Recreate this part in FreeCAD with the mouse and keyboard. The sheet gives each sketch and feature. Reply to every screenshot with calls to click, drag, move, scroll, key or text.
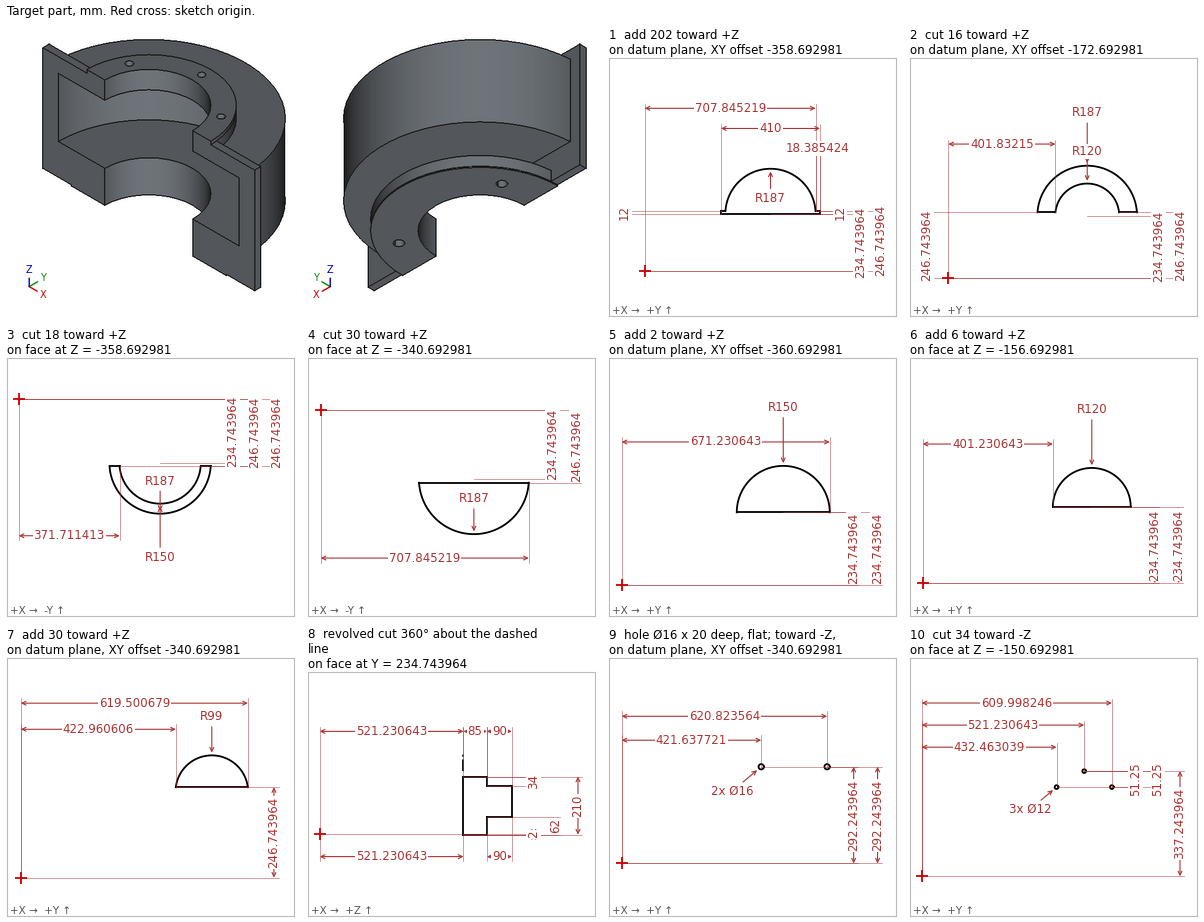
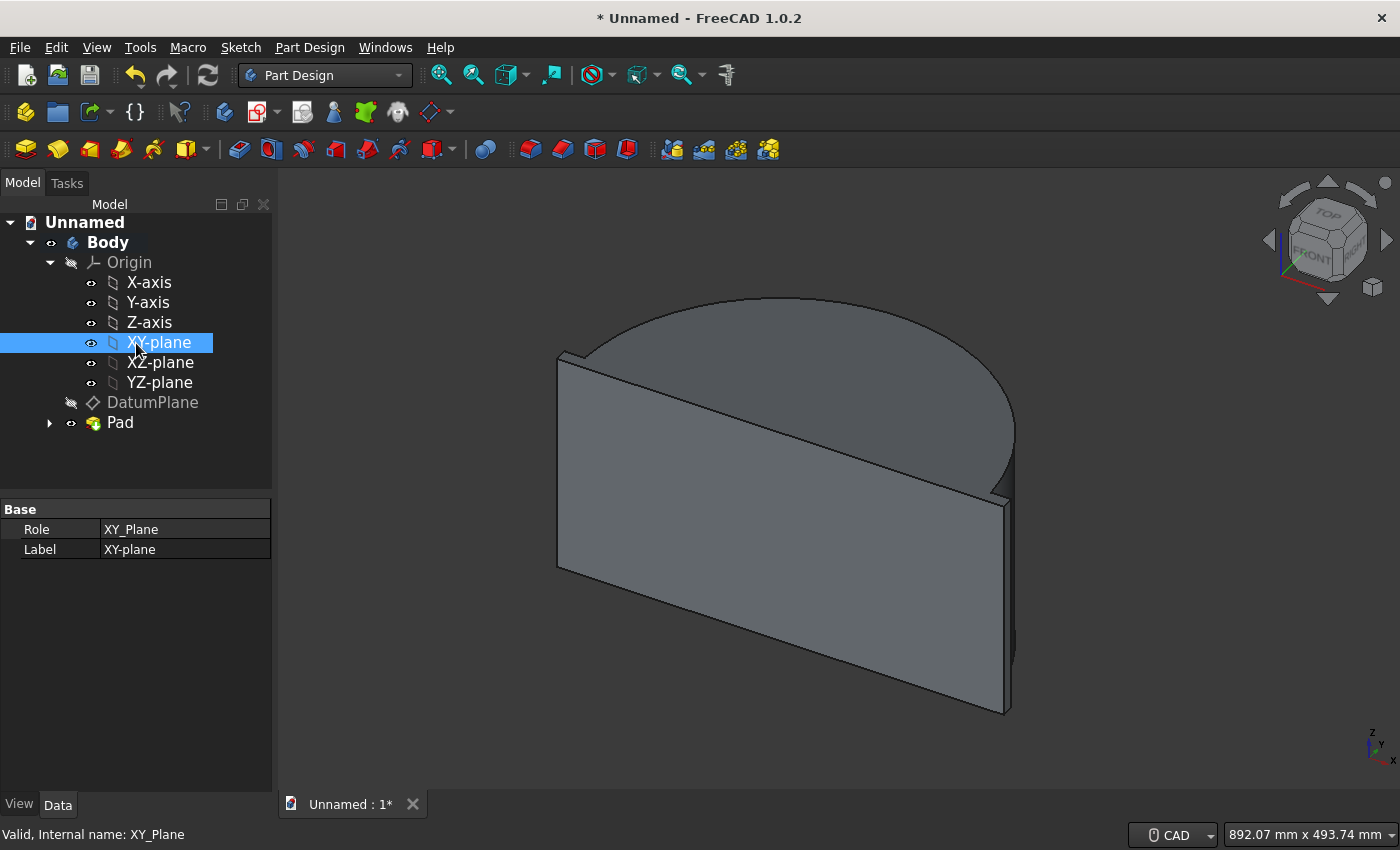
click(430, 112)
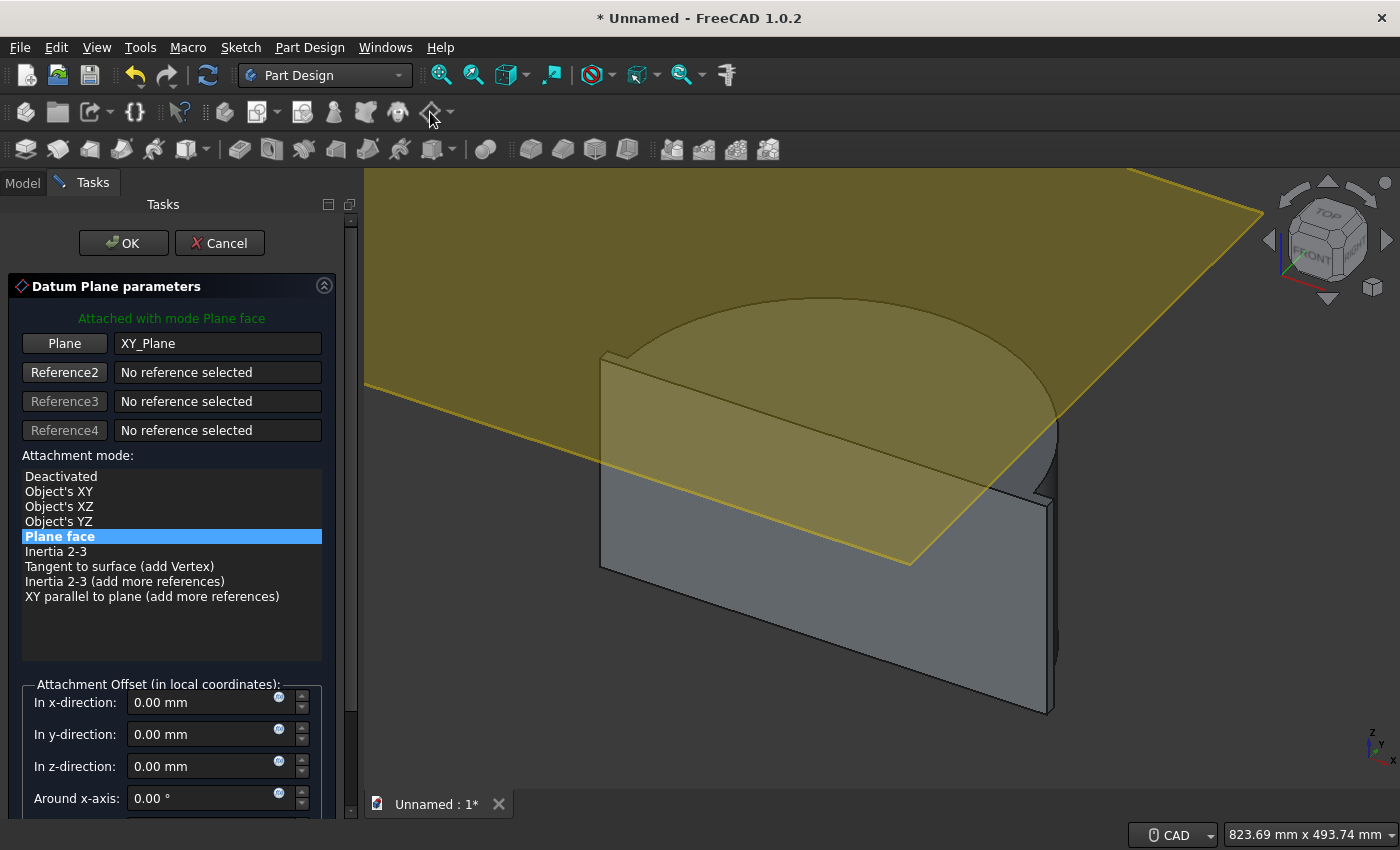
triple_click(210, 766)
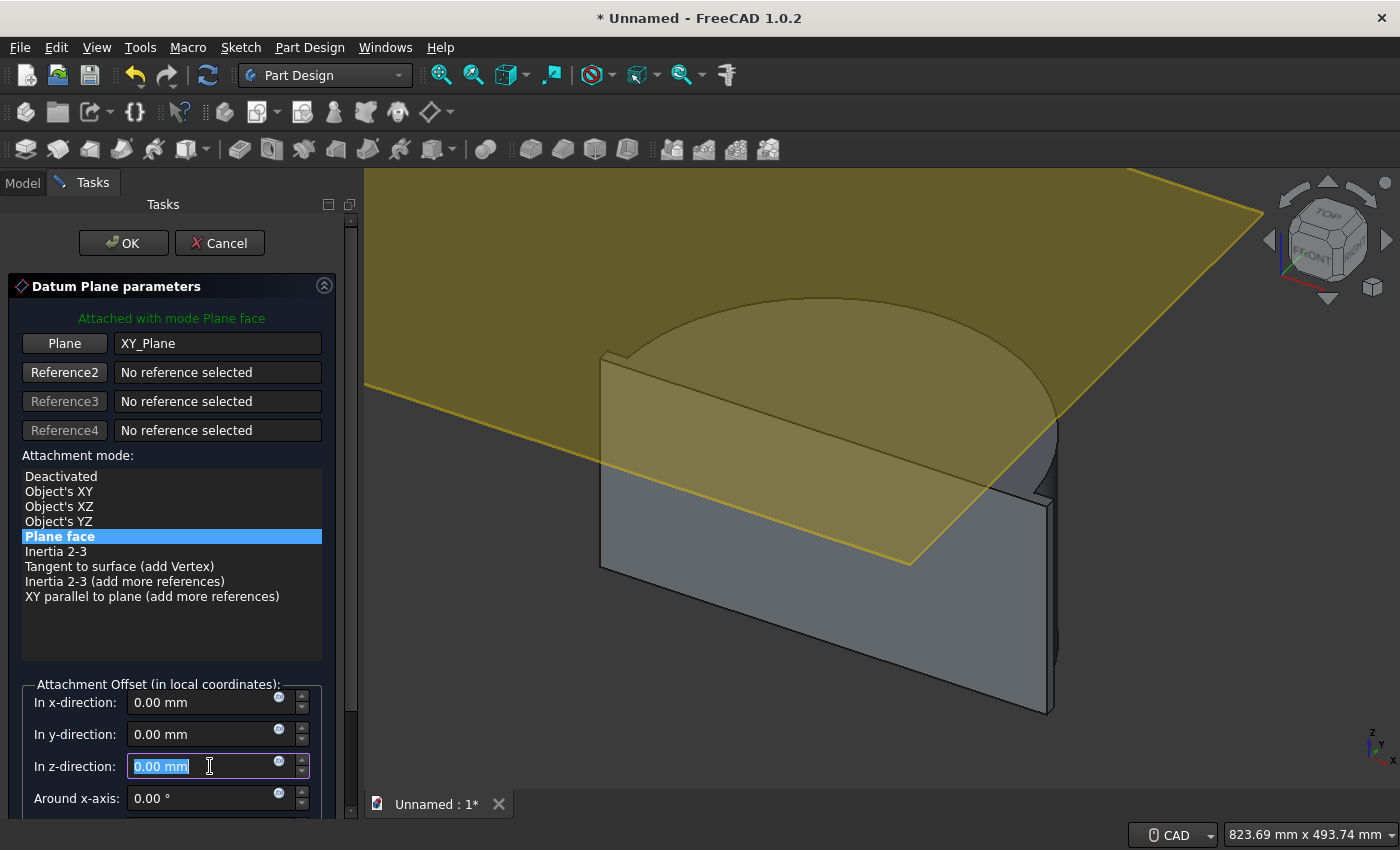
text(-172.692981)
key(Tab)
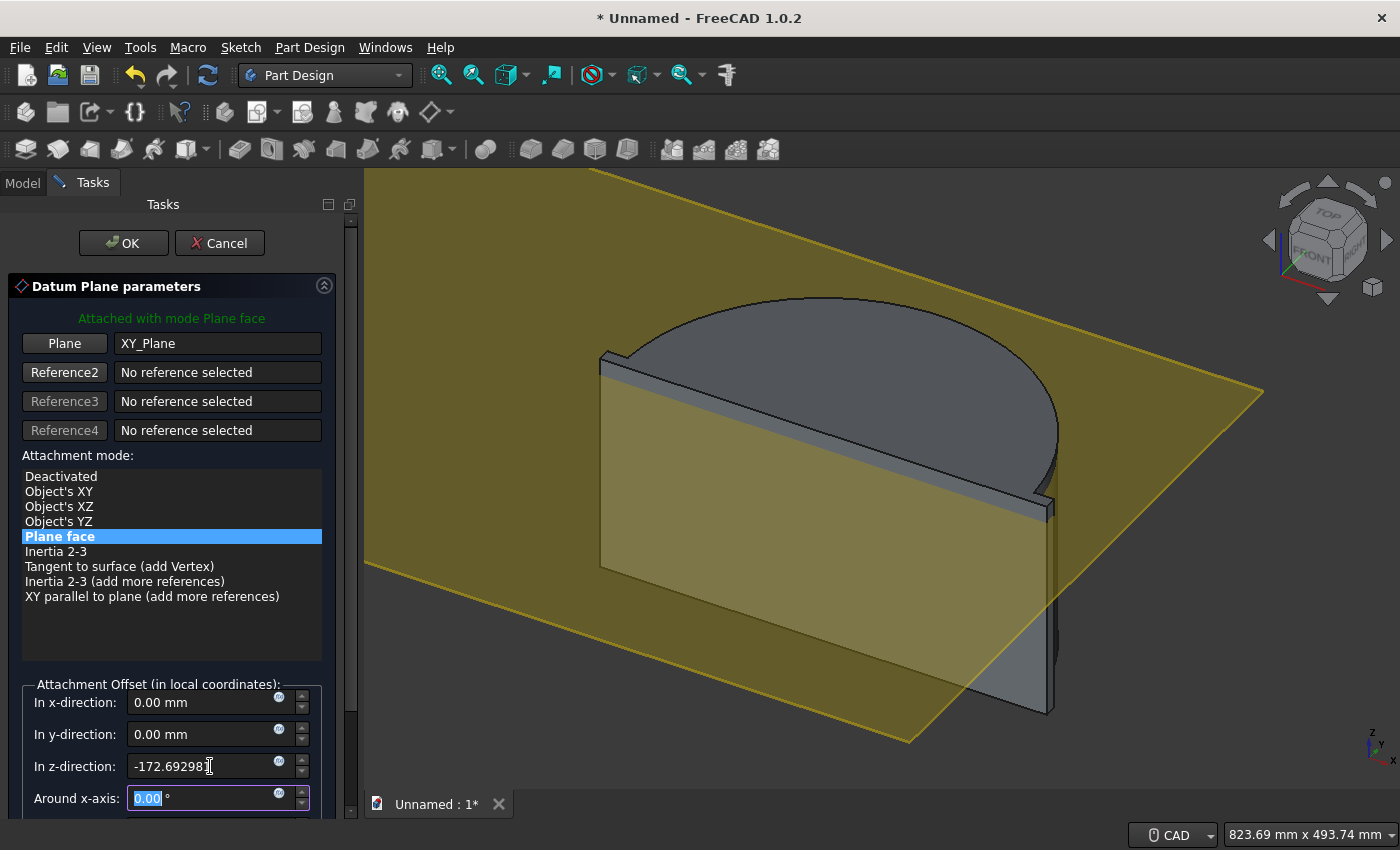
click(124, 243)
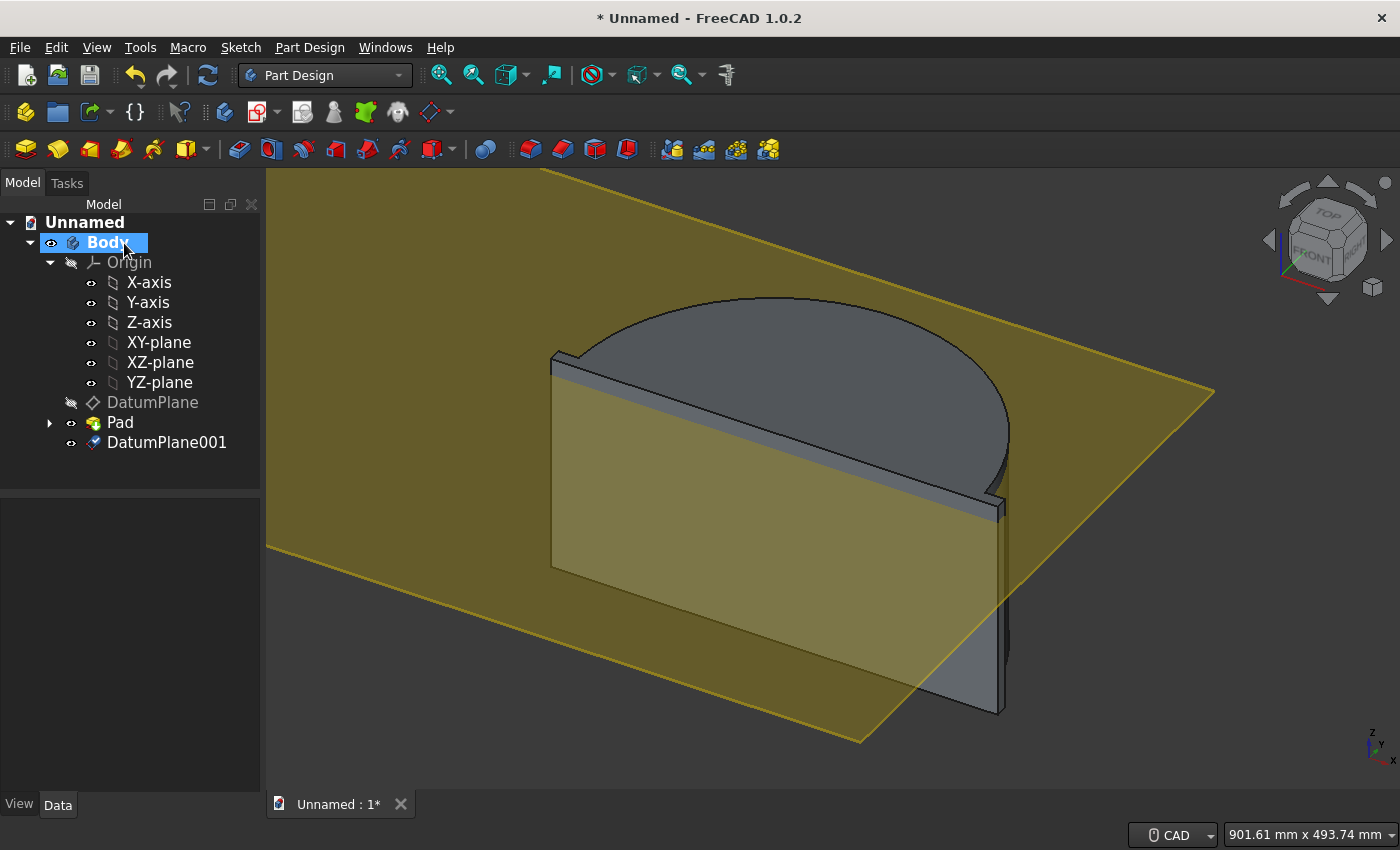
click(116, 443)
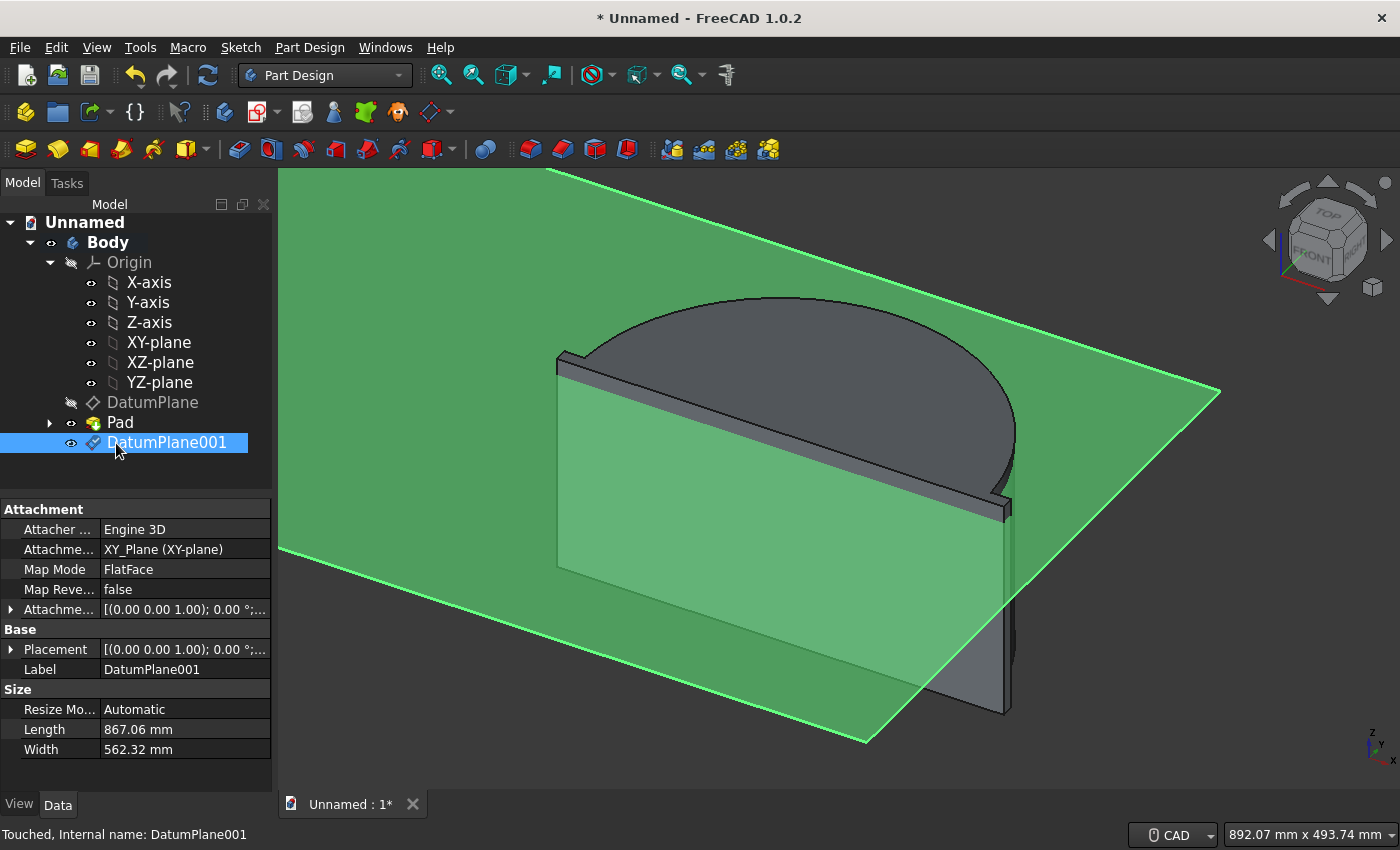
click(258, 112)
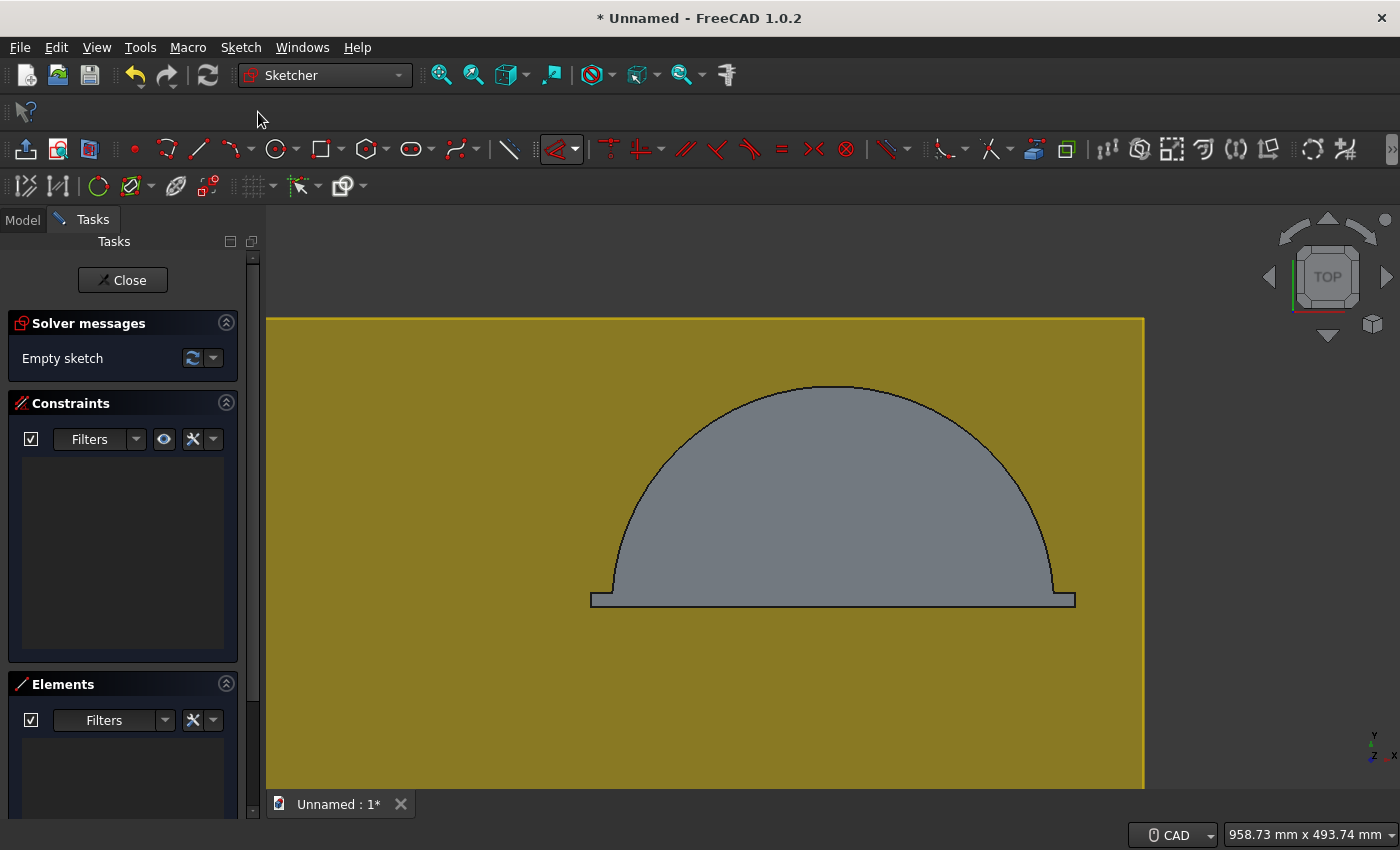
key(q)
key(s)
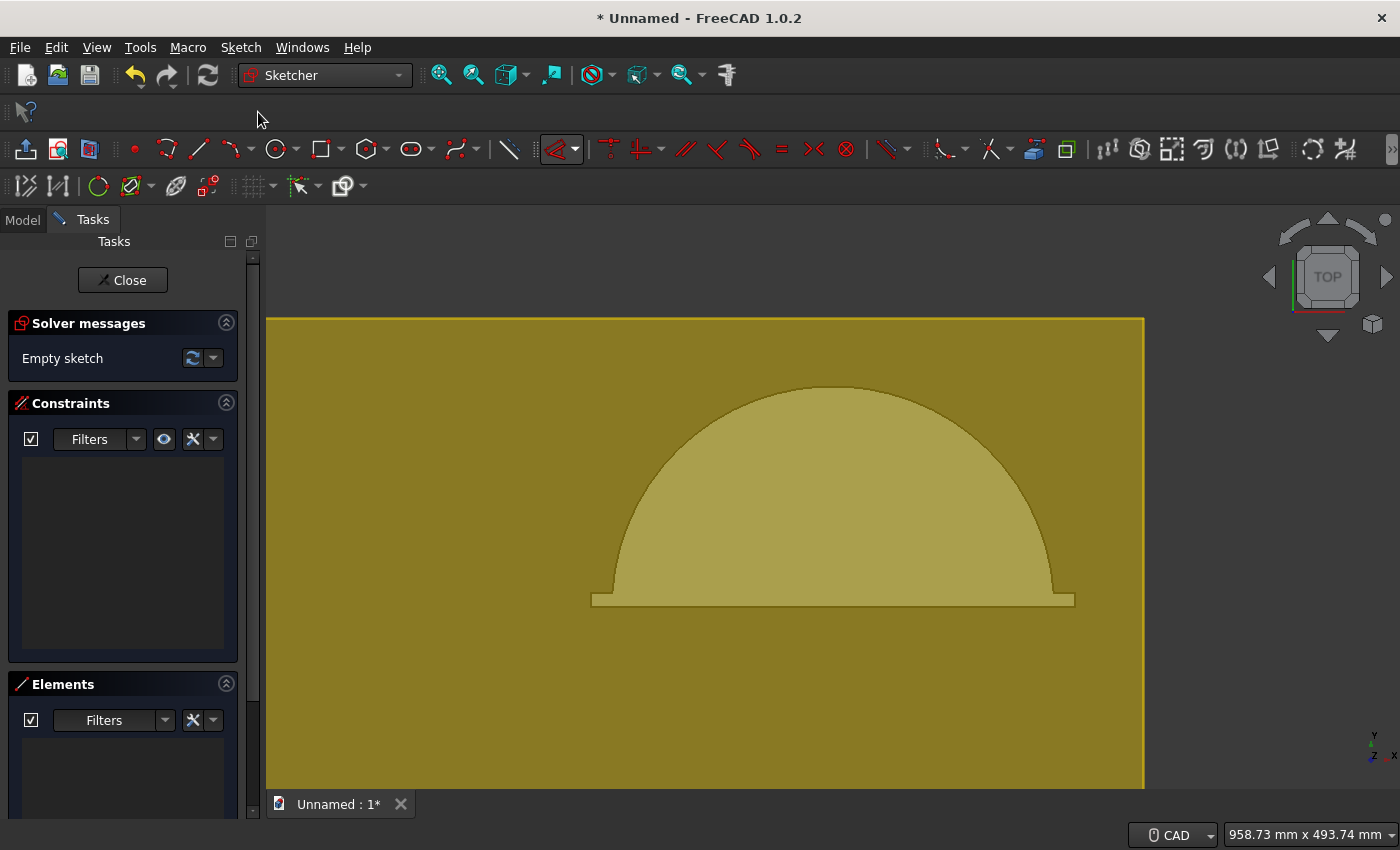
scroll(1028, 233, down, 2)